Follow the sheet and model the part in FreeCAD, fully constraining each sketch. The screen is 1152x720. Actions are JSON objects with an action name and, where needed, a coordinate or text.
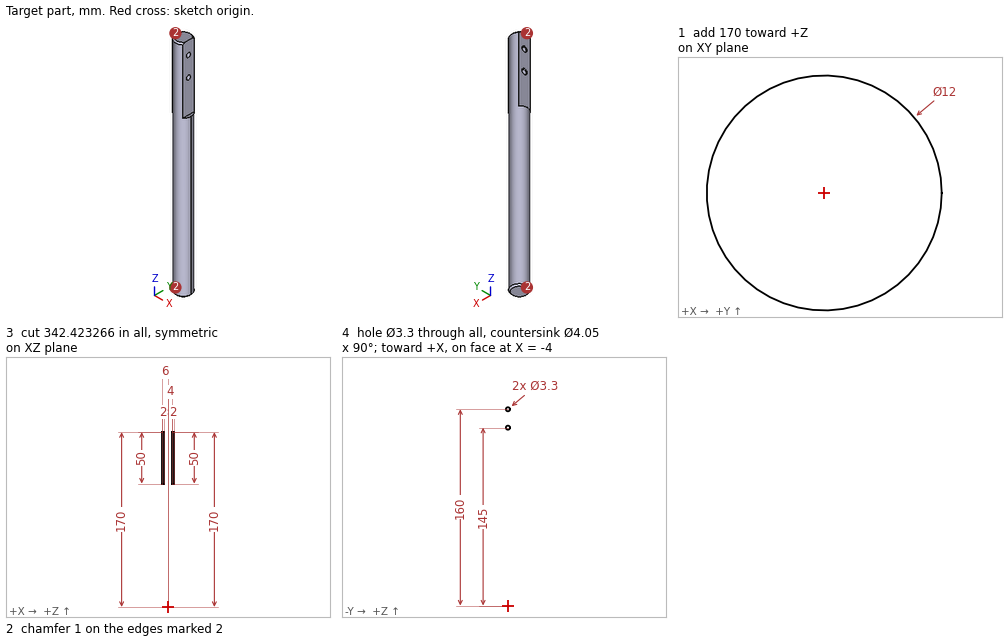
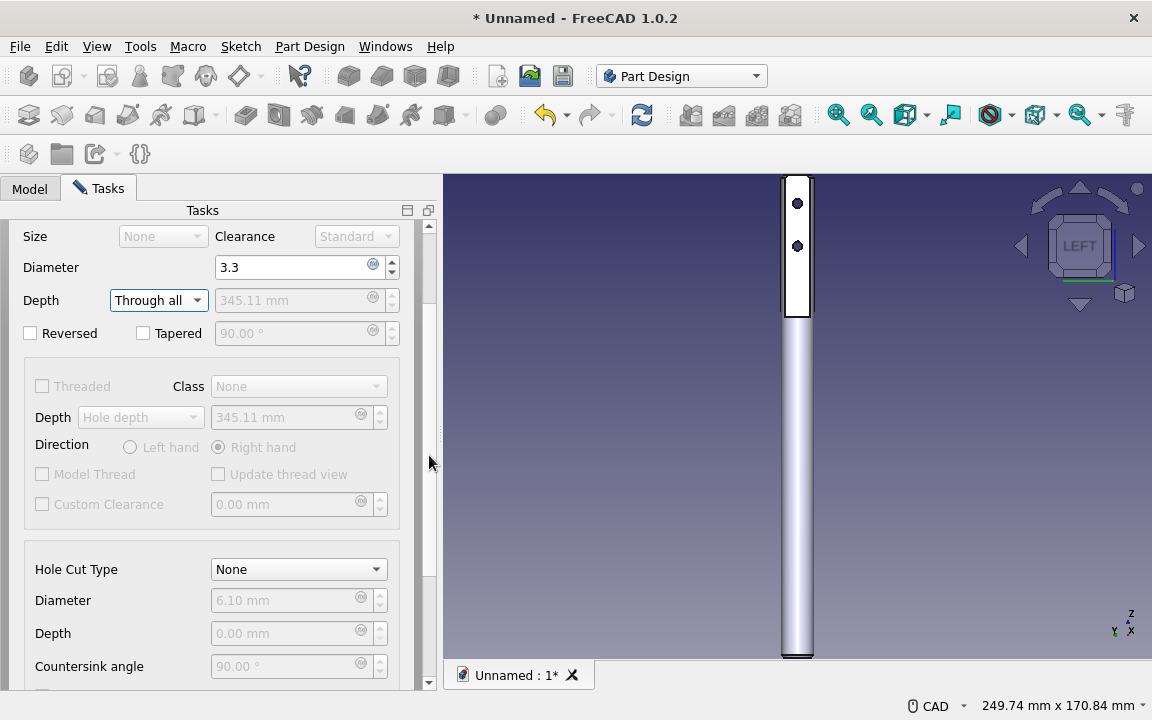
{"action": "left_click", "coordinate": [300, 570]}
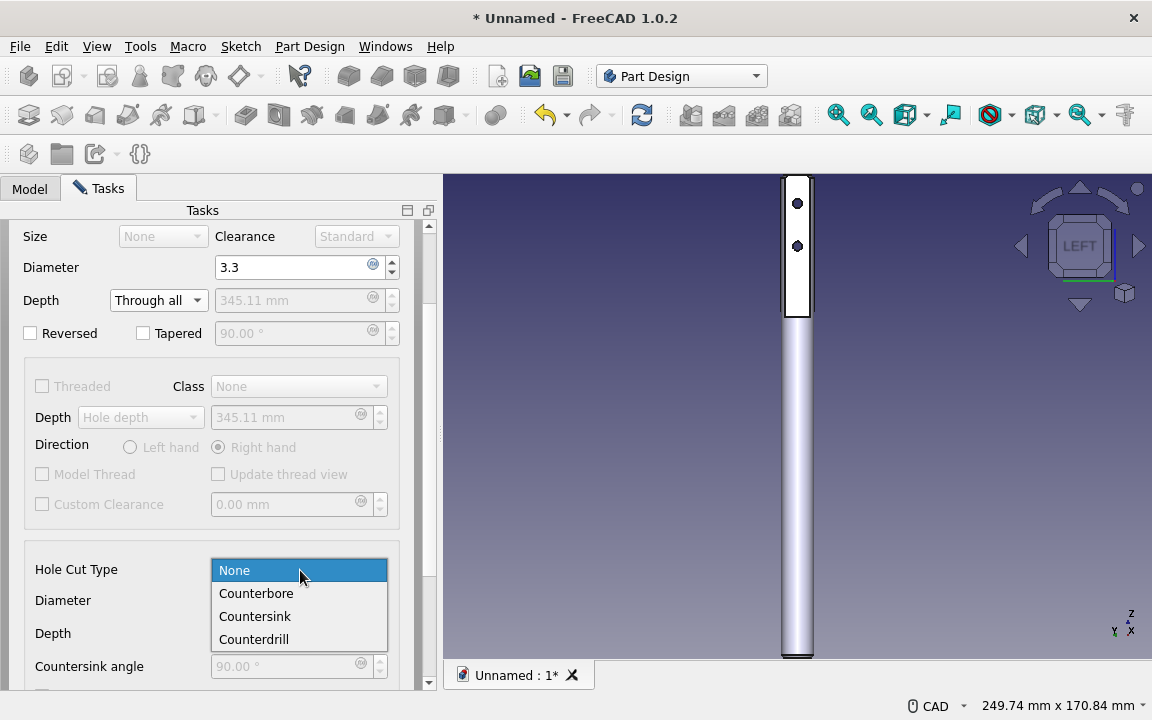
{"action": "left_click", "coordinate": [298, 616]}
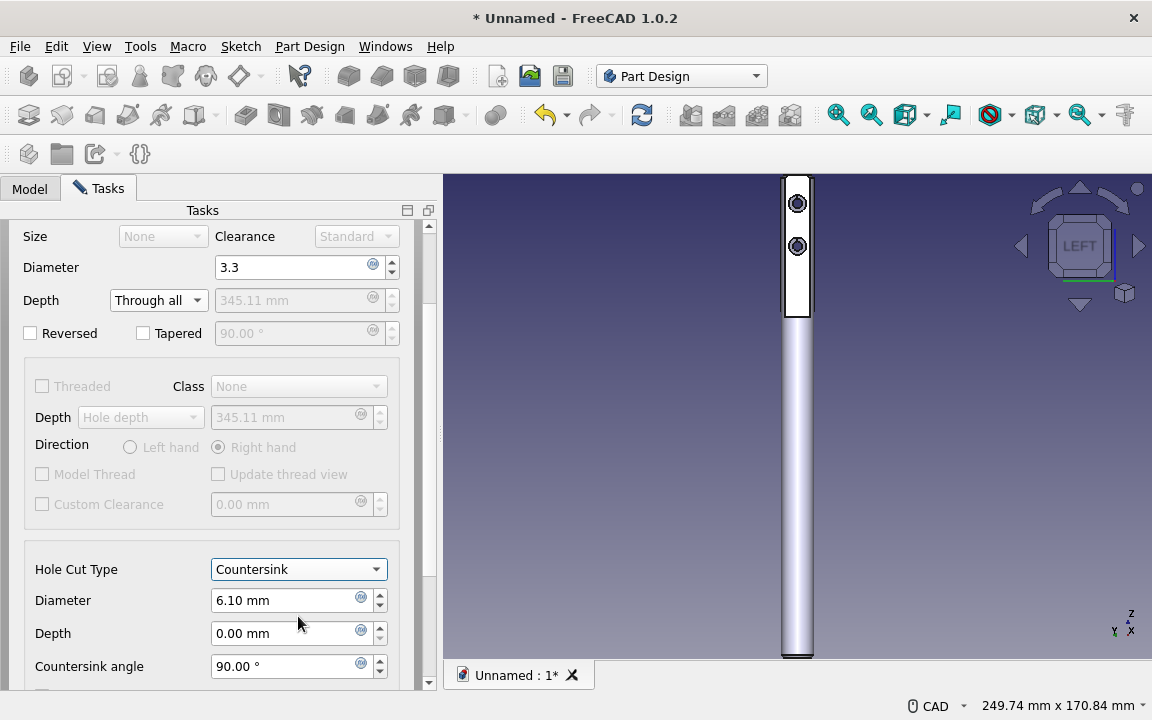
{"action": "triple_click", "coordinate": [292, 600]}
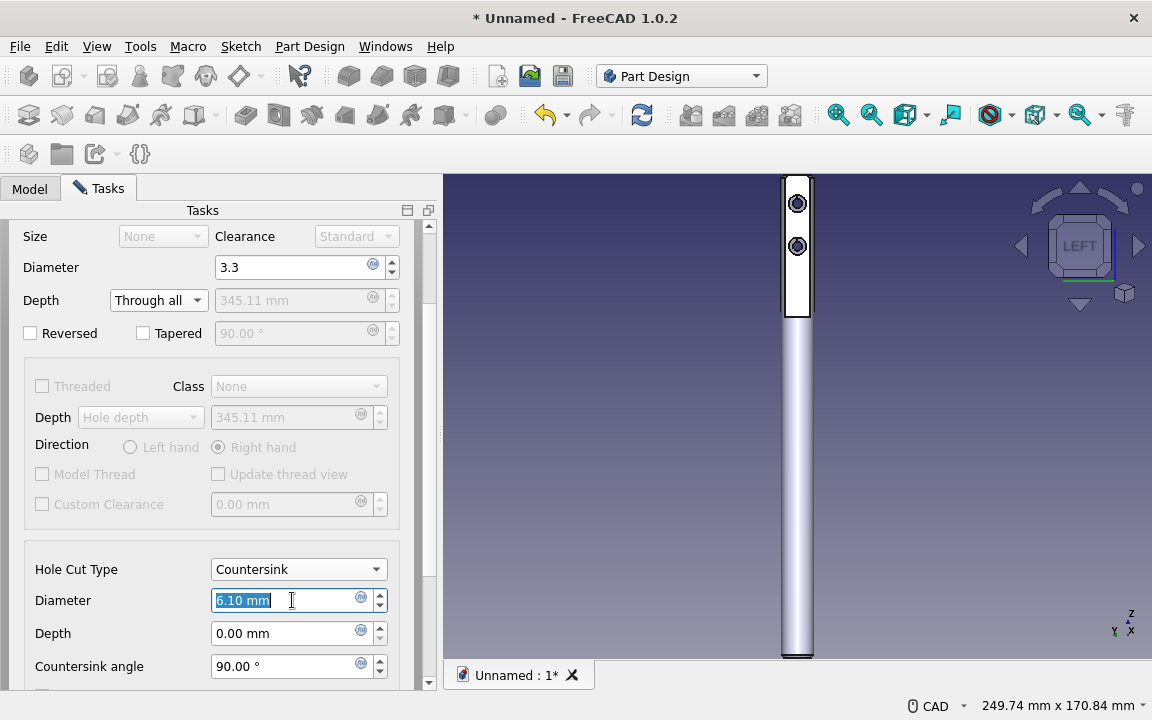
{"action": "type", "text": "4.05"}
{"action": "key", "text": "Tab"}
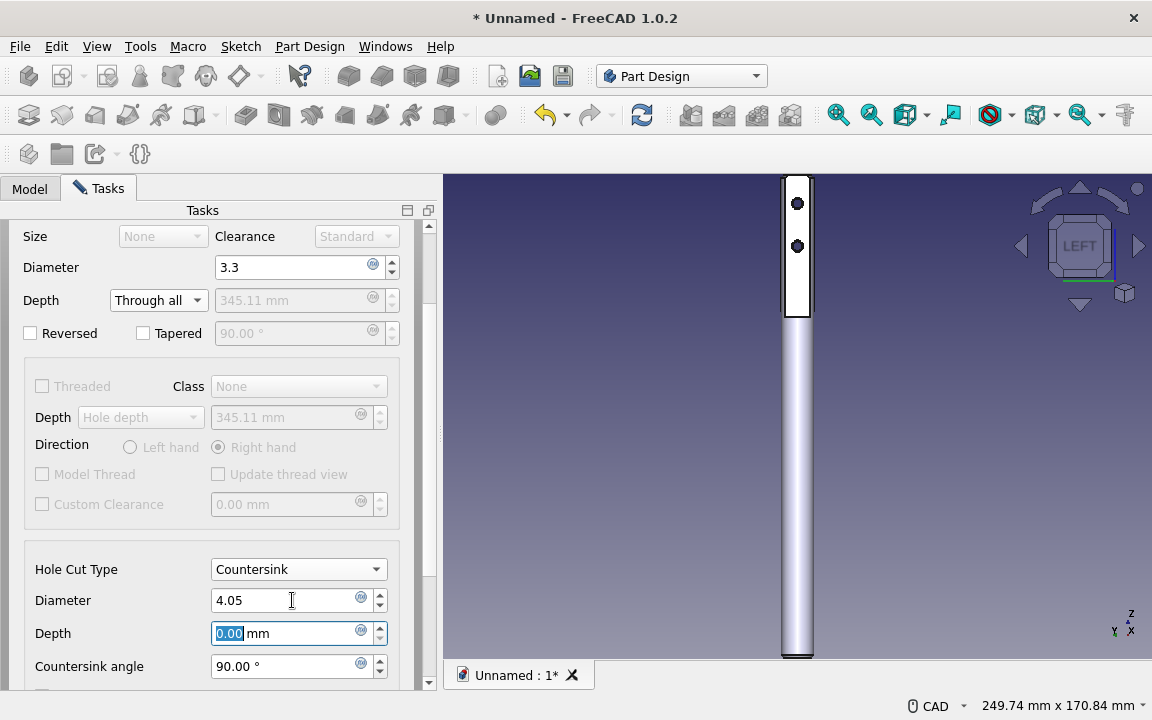
{"action": "scroll", "coordinate": [429, 455], "scroll_direction": "up", "scroll_amount": 3}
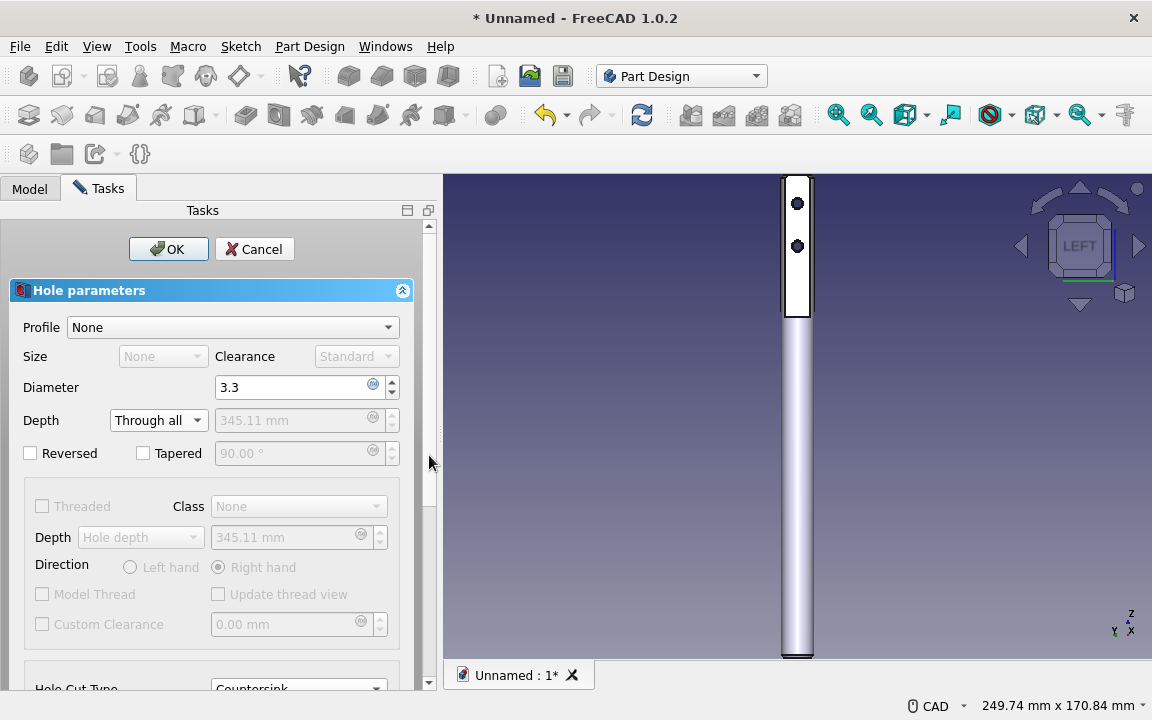
{"action": "left_click", "coordinate": [169, 249]}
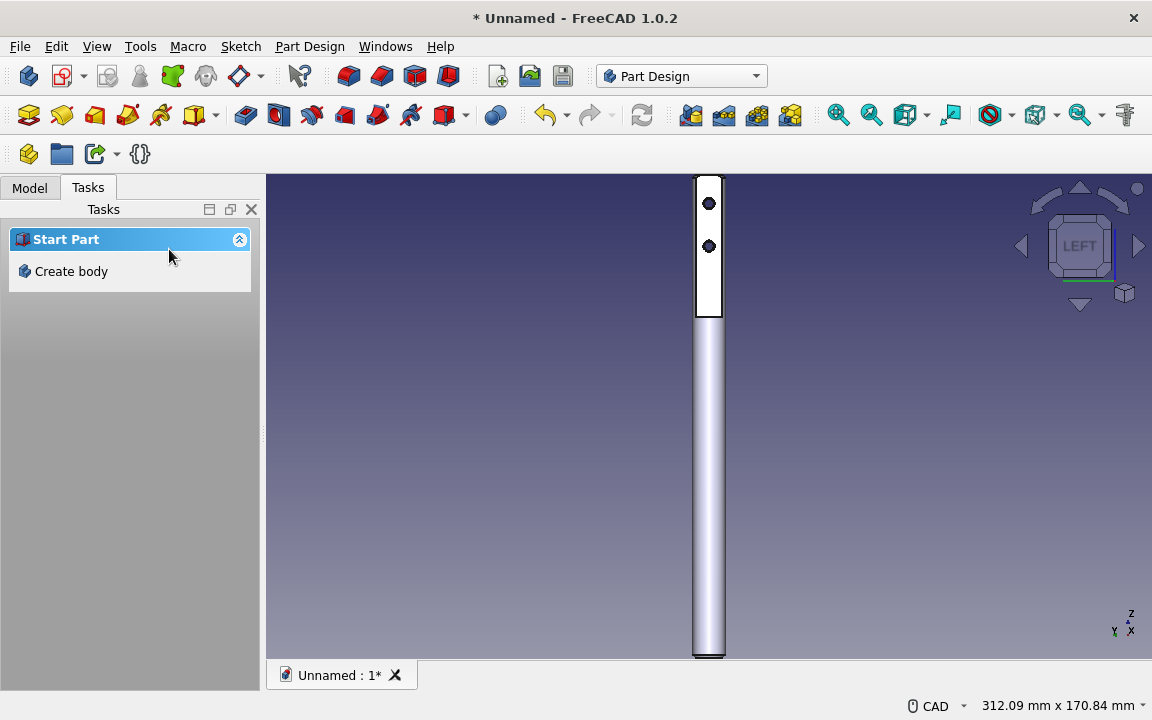
{"action": "key", "text": "0"}